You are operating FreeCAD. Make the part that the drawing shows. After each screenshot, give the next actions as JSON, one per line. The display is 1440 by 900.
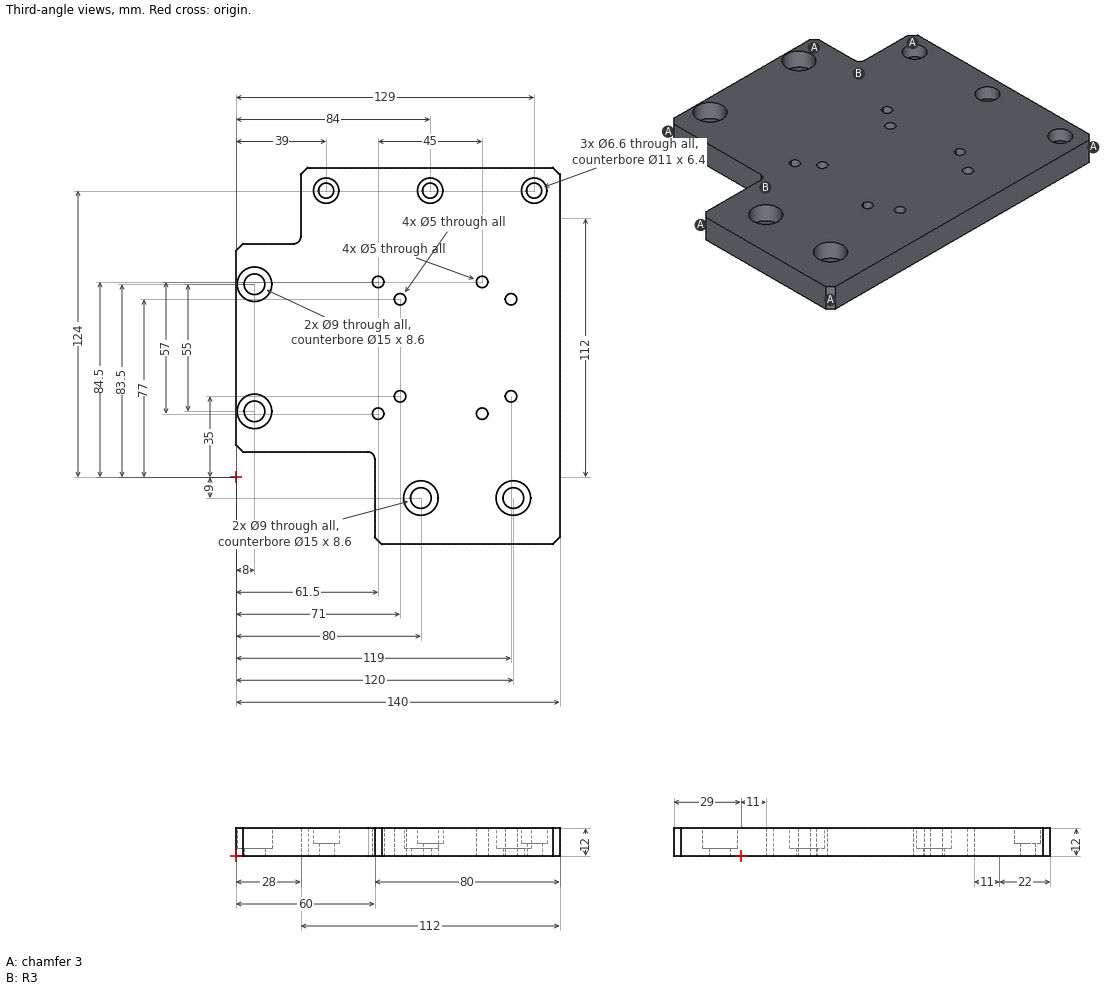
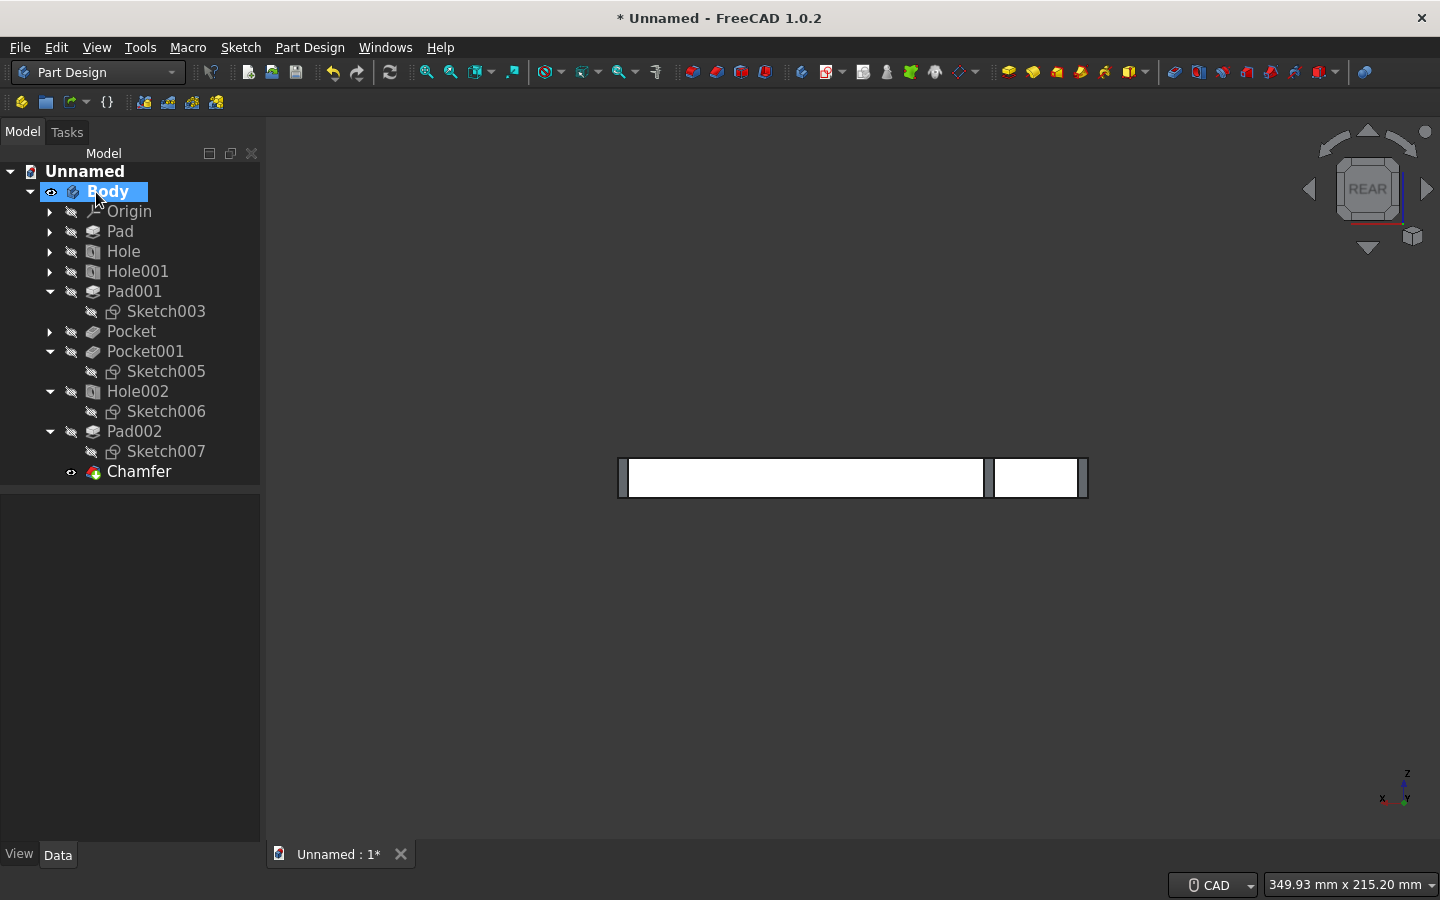
{"action": "key", "text": "v f"}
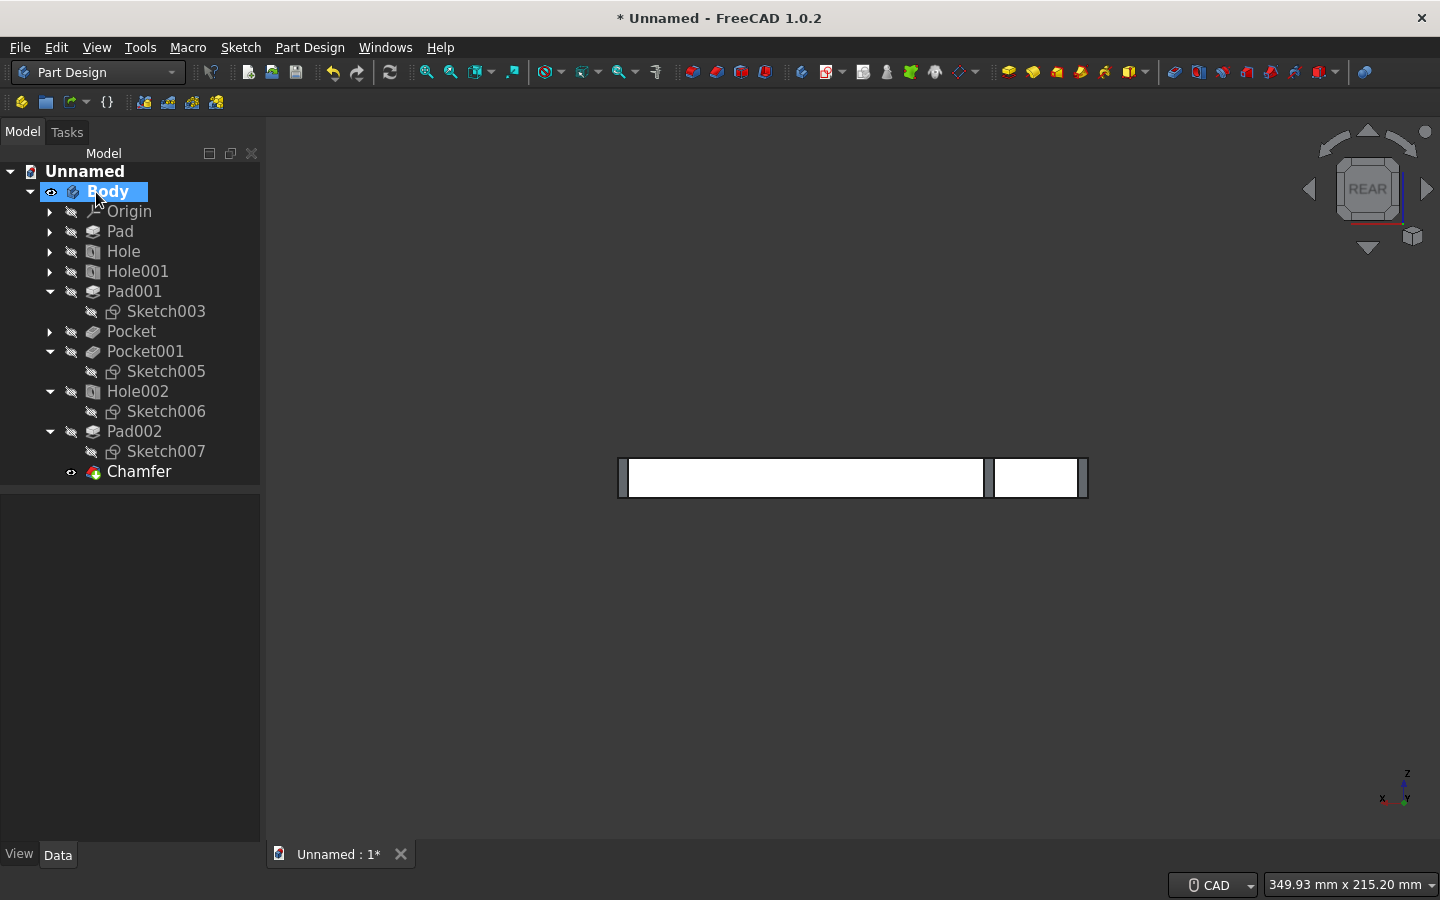
{"action": "key", "text": "0"}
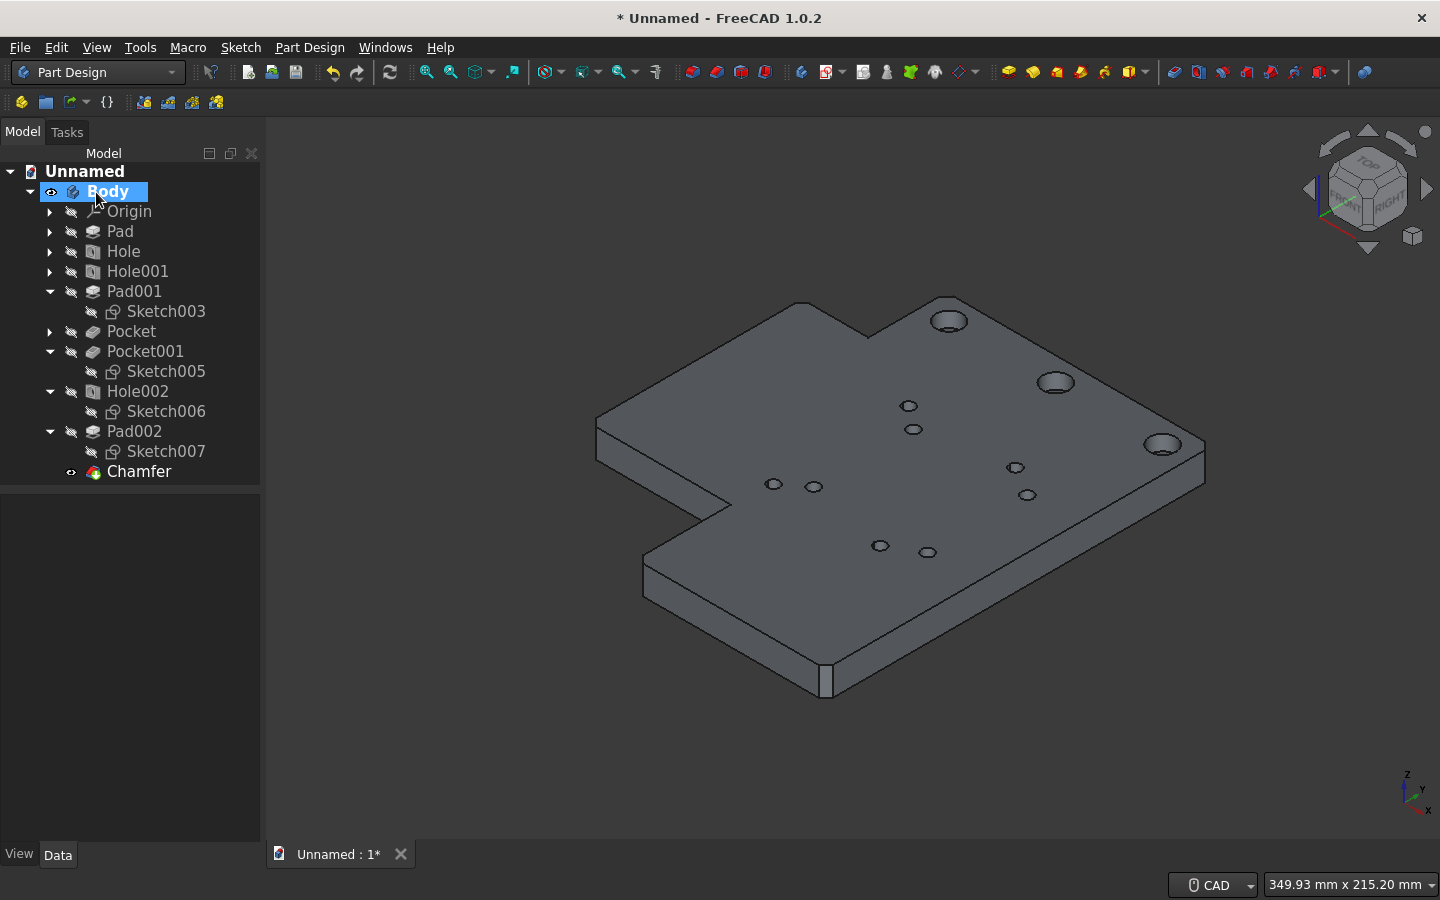
{"action": "key", "text": "2"}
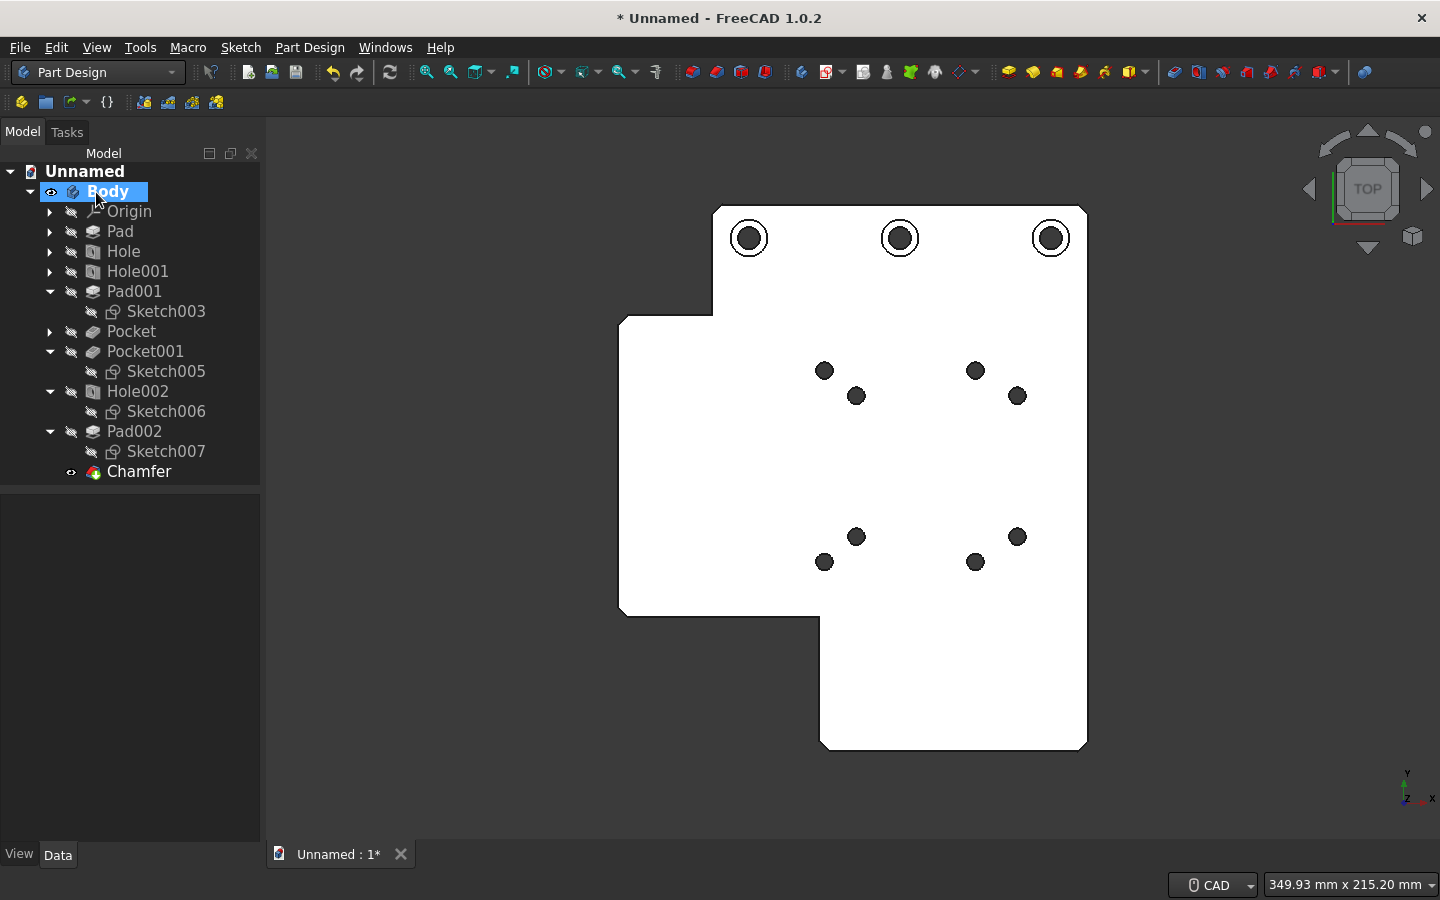
{"action": "key", "text": "1"}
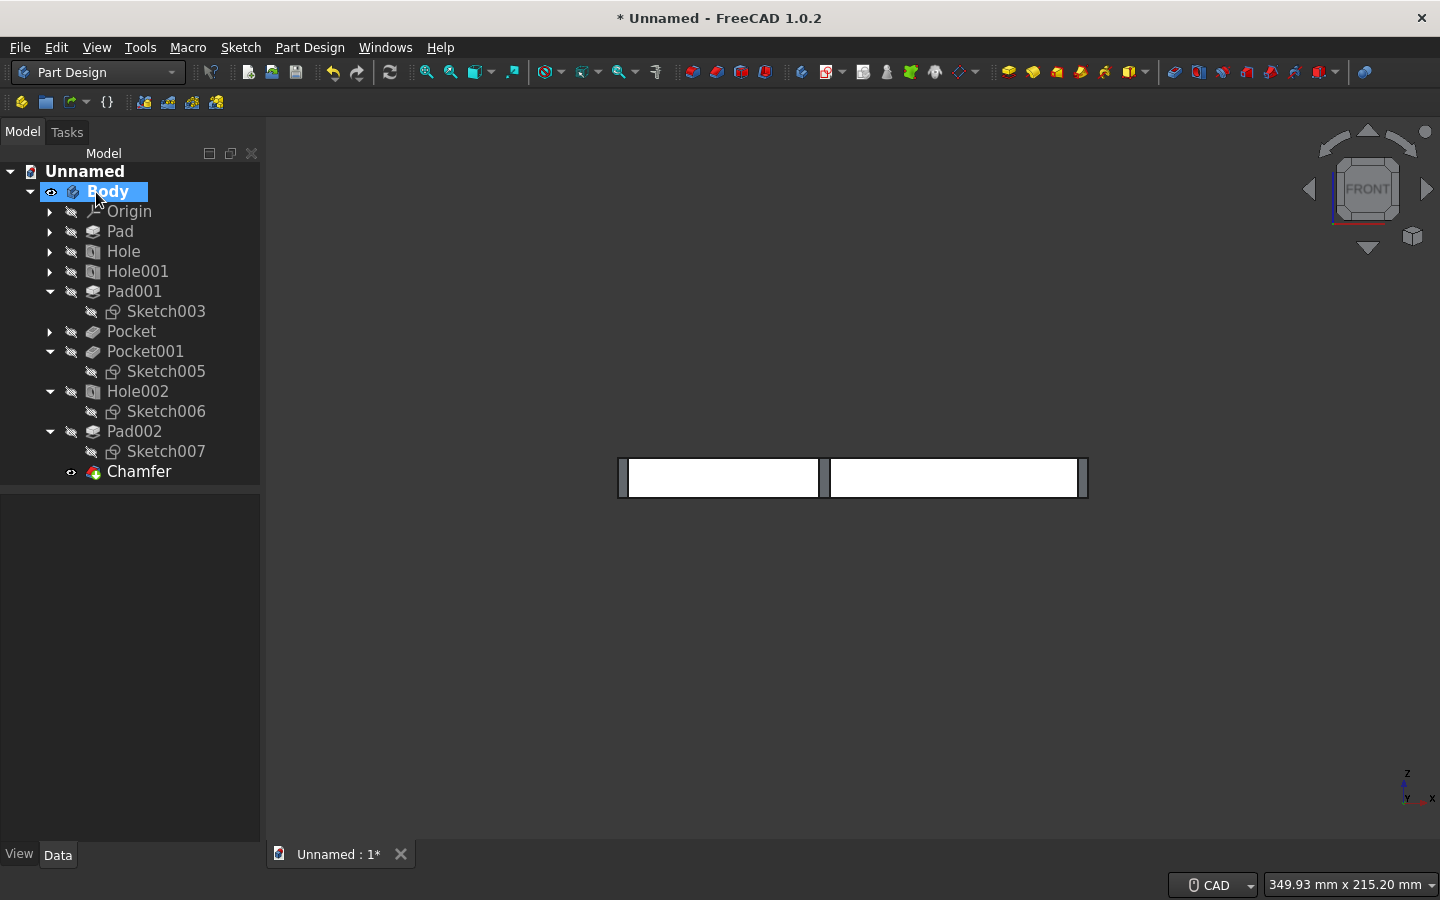
{"action": "left_click", "coordinate": [428, 72]}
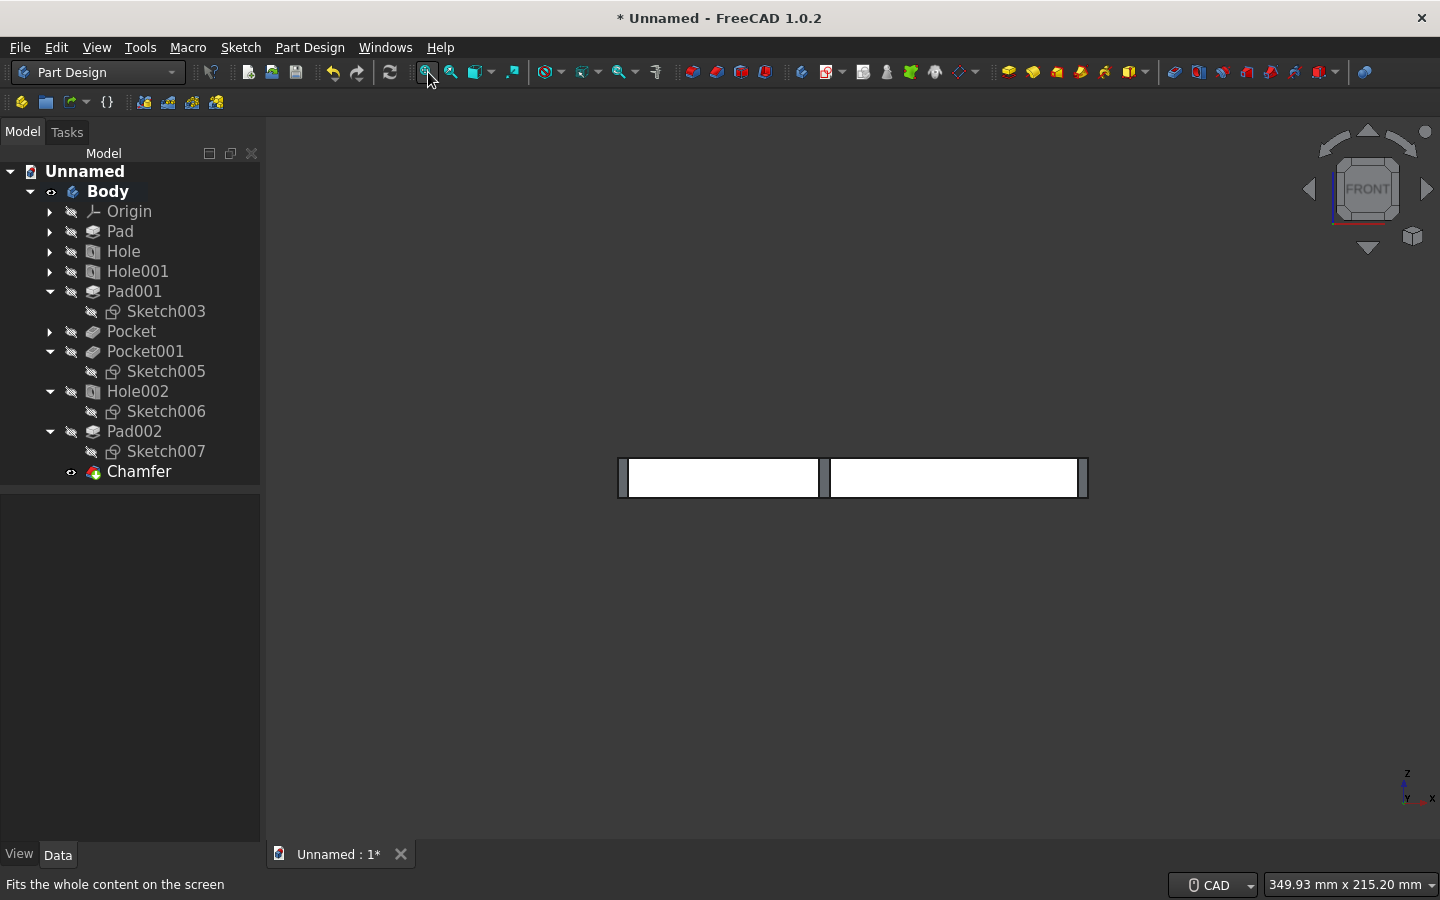
{"action": "key", "text": "3"}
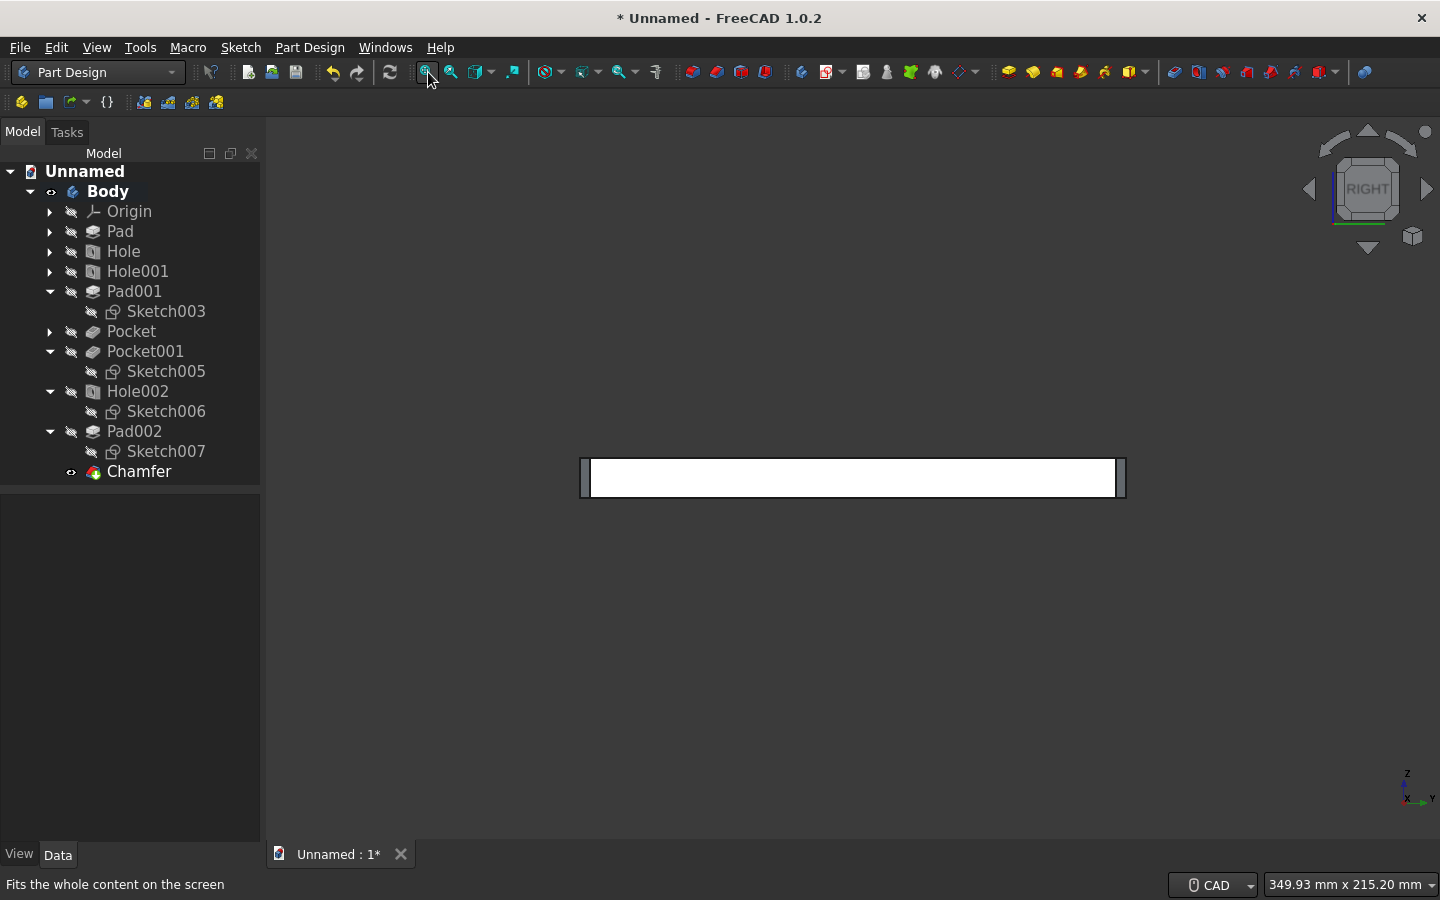
{"action": "key", "text": "5"}